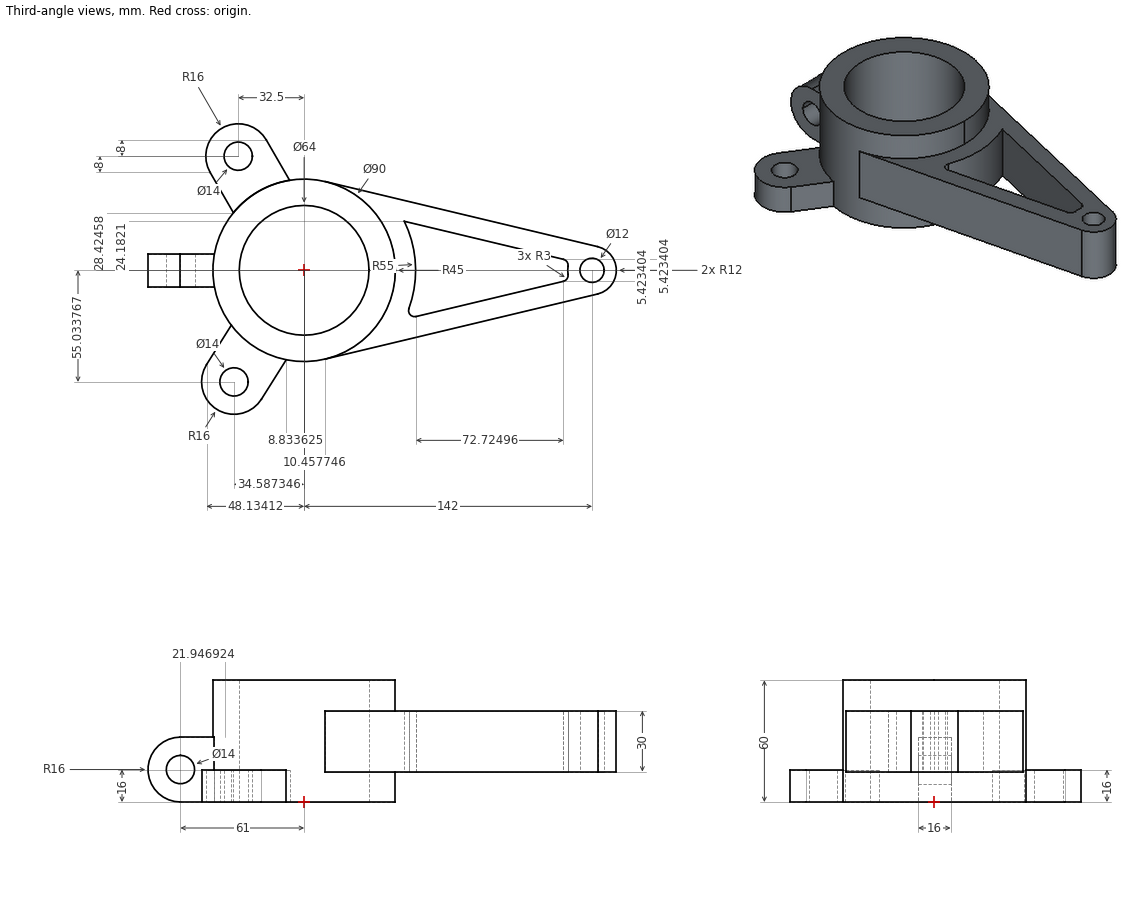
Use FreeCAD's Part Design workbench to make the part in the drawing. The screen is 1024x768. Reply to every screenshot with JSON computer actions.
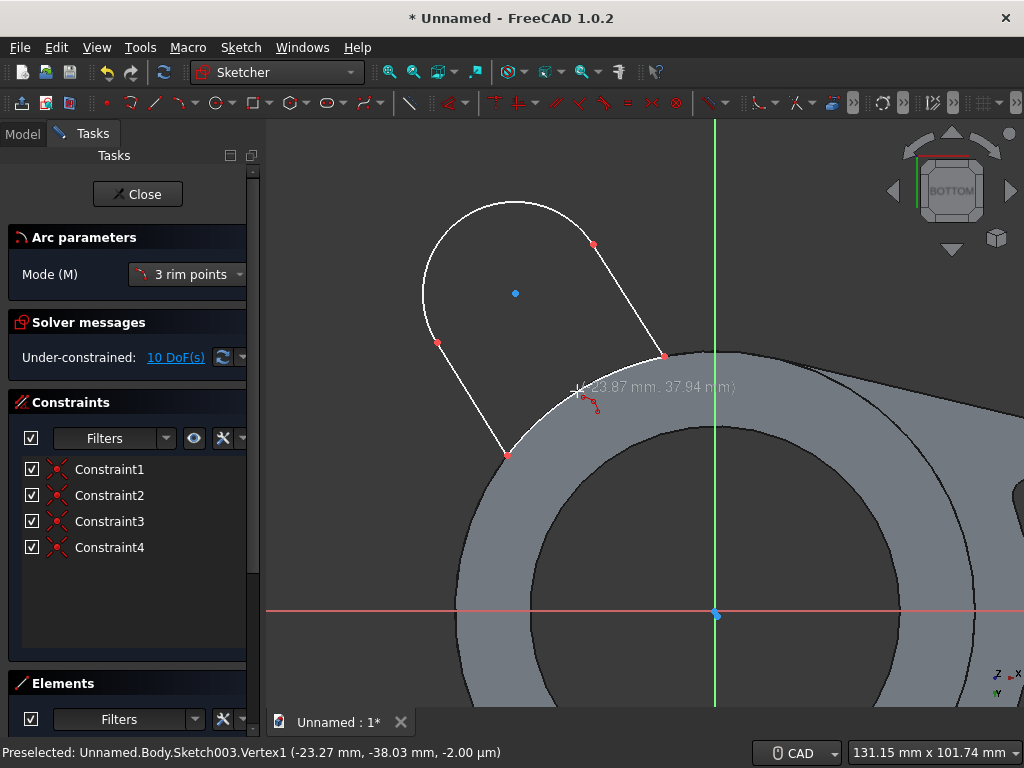
{"action": "left_click", "coordinate": [216, 104]}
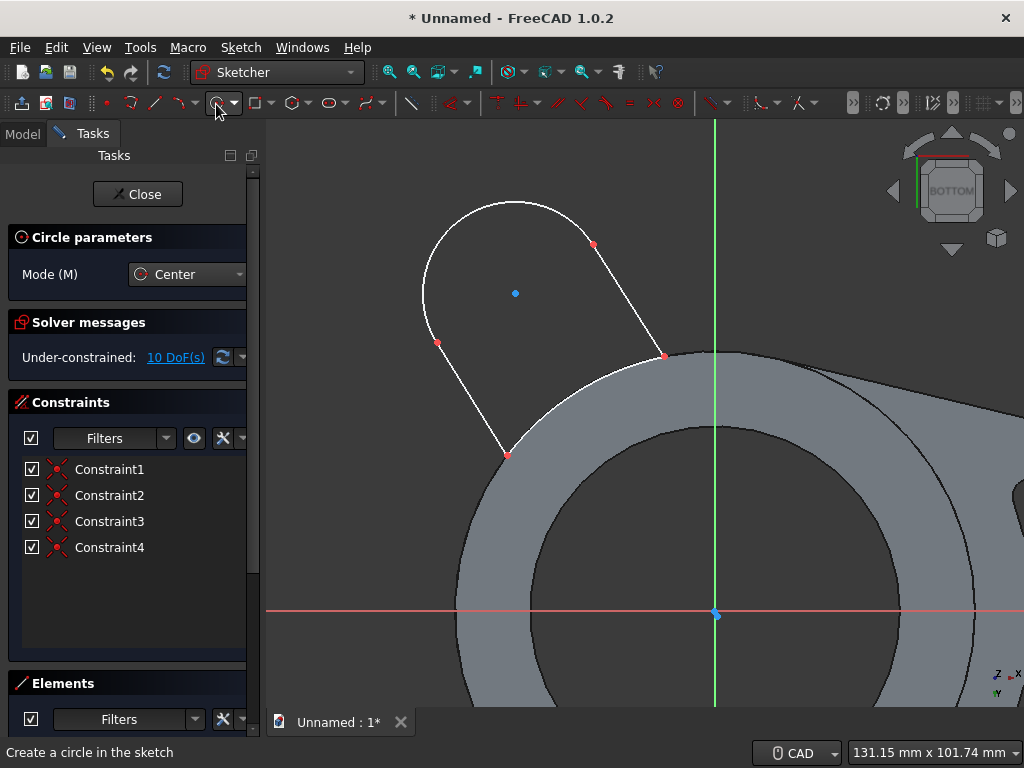
{"action": "left_click", "coordinate": [515, 293]}
{"action": "left_click", "coordinate": [544, 265]}
{"action": "key", "text": "Escape"}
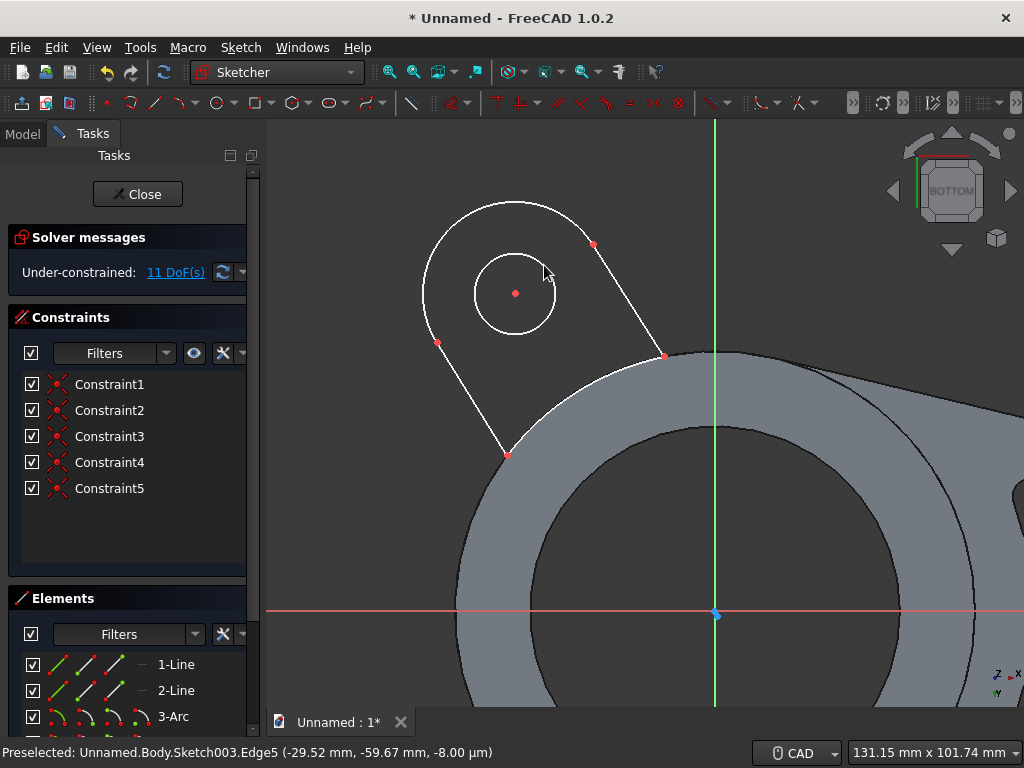
{"action": "left_click", "coordinate": [486, 422]}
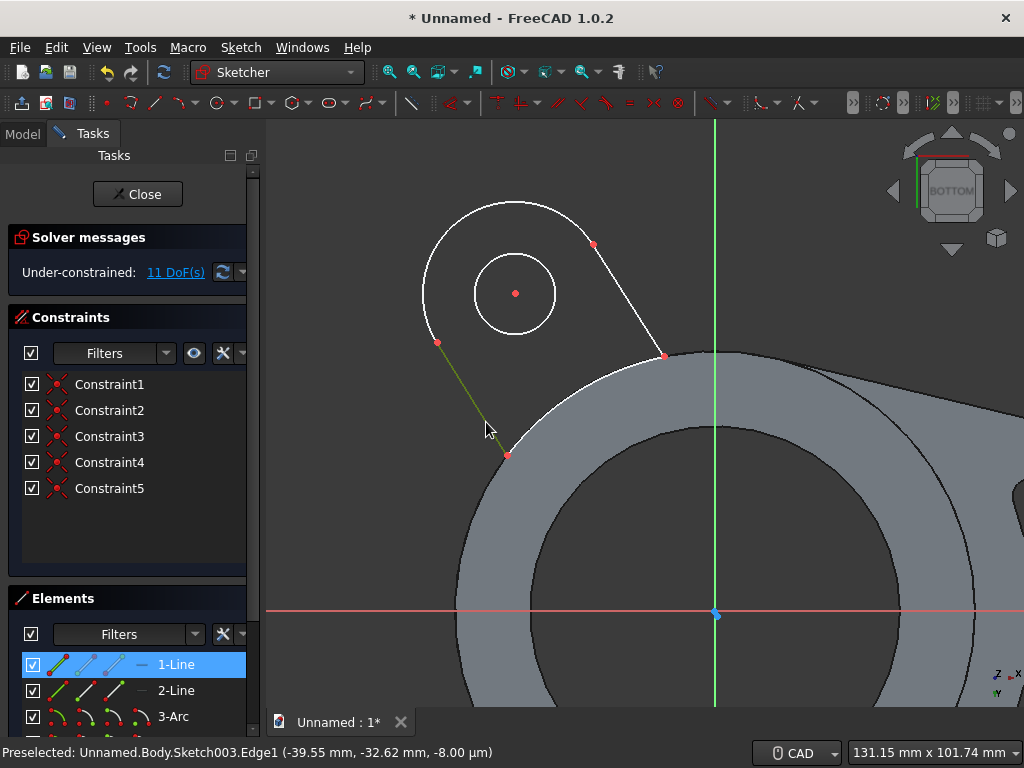
{"action": "left_click", "coordinate": [521, 202]}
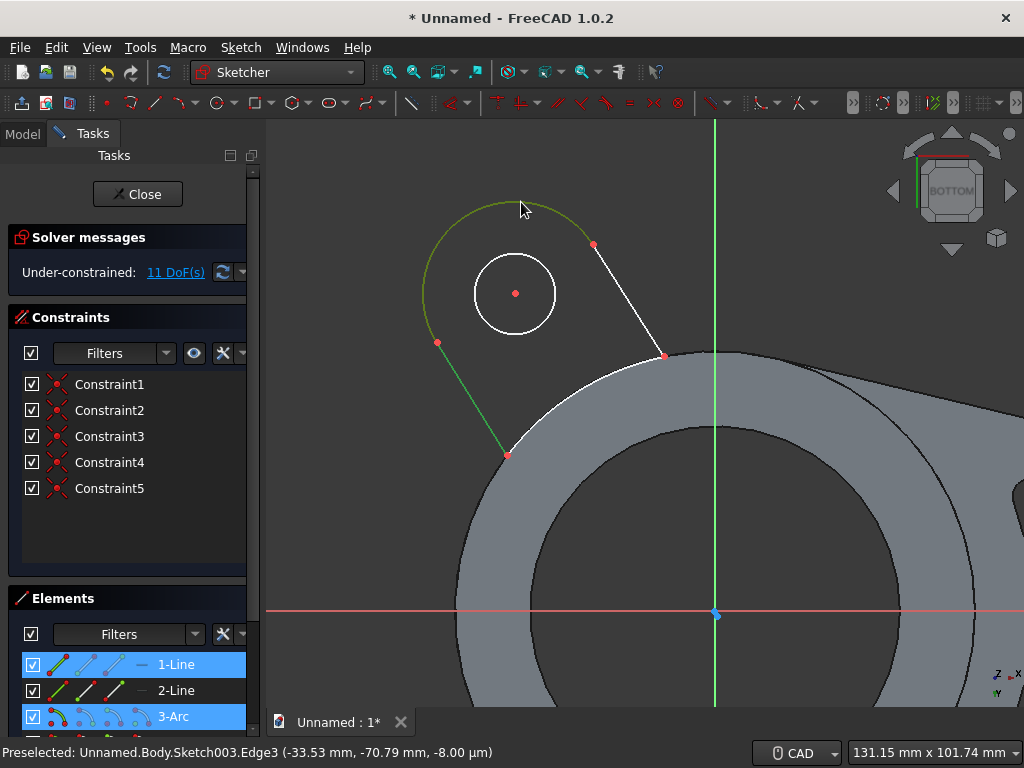
{"action": "key", "text": "t"}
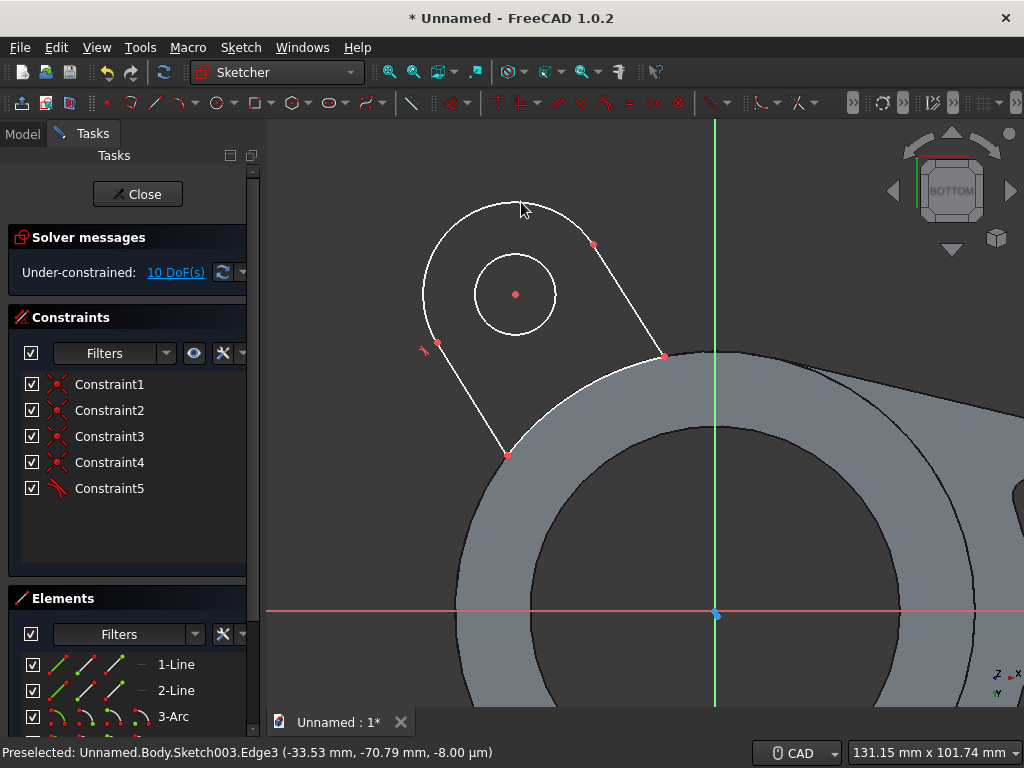
{"action": "left_click", "coordinate": [614, 279]}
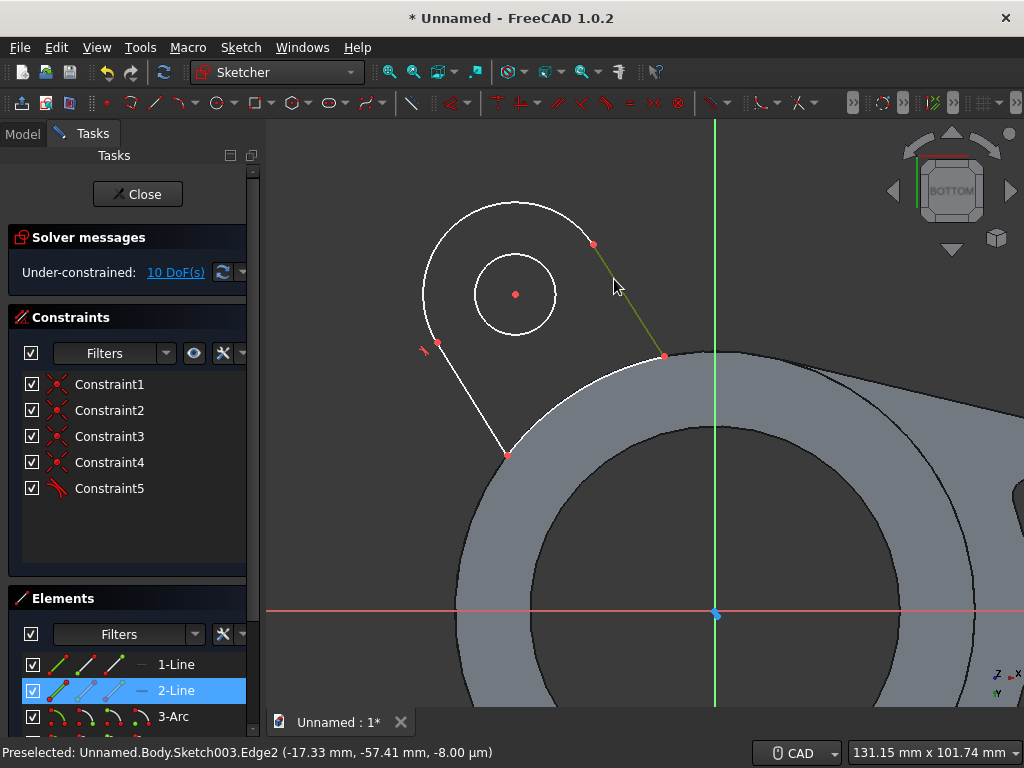
{"action": "left_click", "coordinate": [521, 203]}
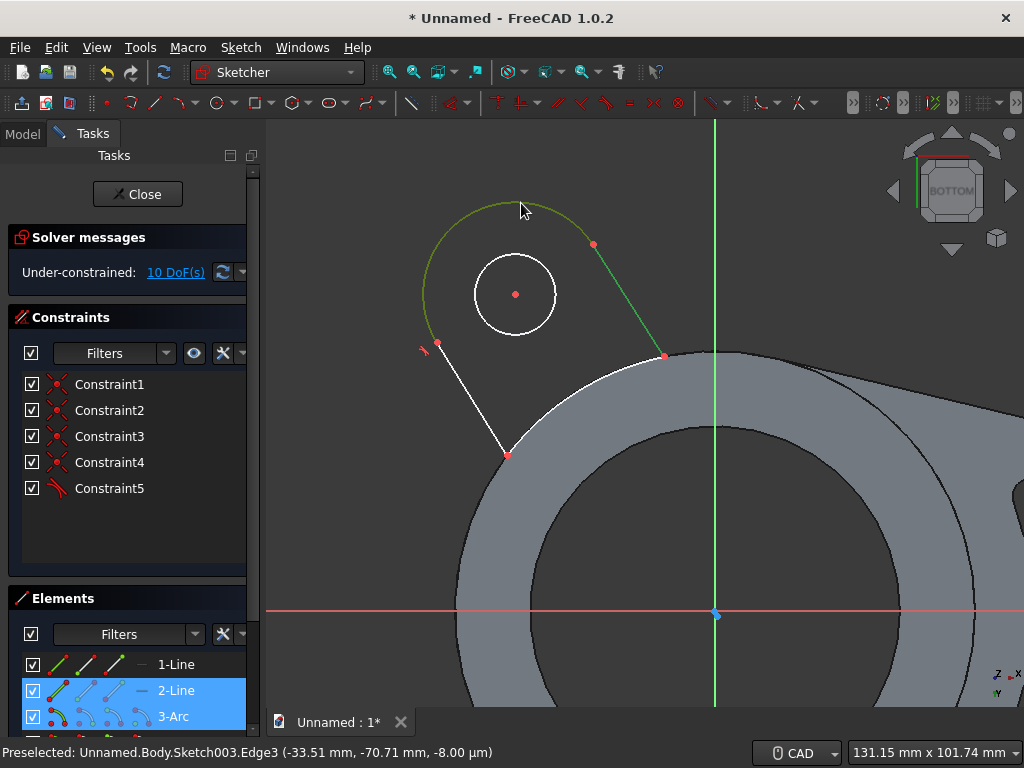
{"action": "left_click", "coordinate": [606, 104]}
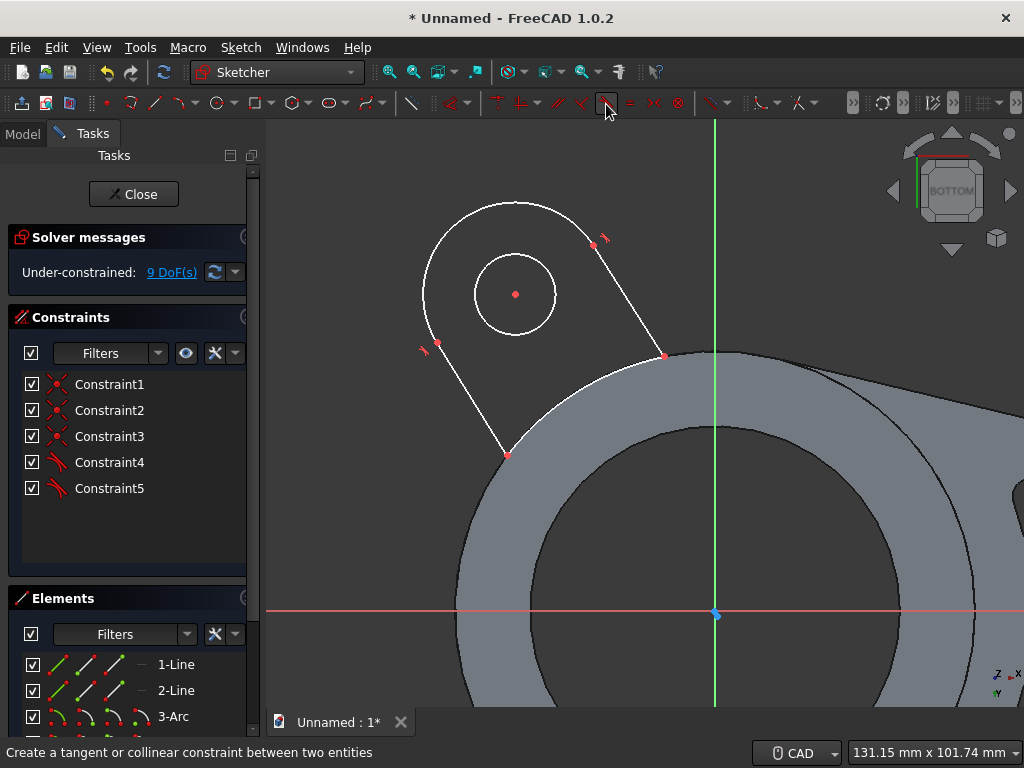
{"action": "left_click_drag", "start_coordinate": [705, 601], "coordinate": [728, 626]}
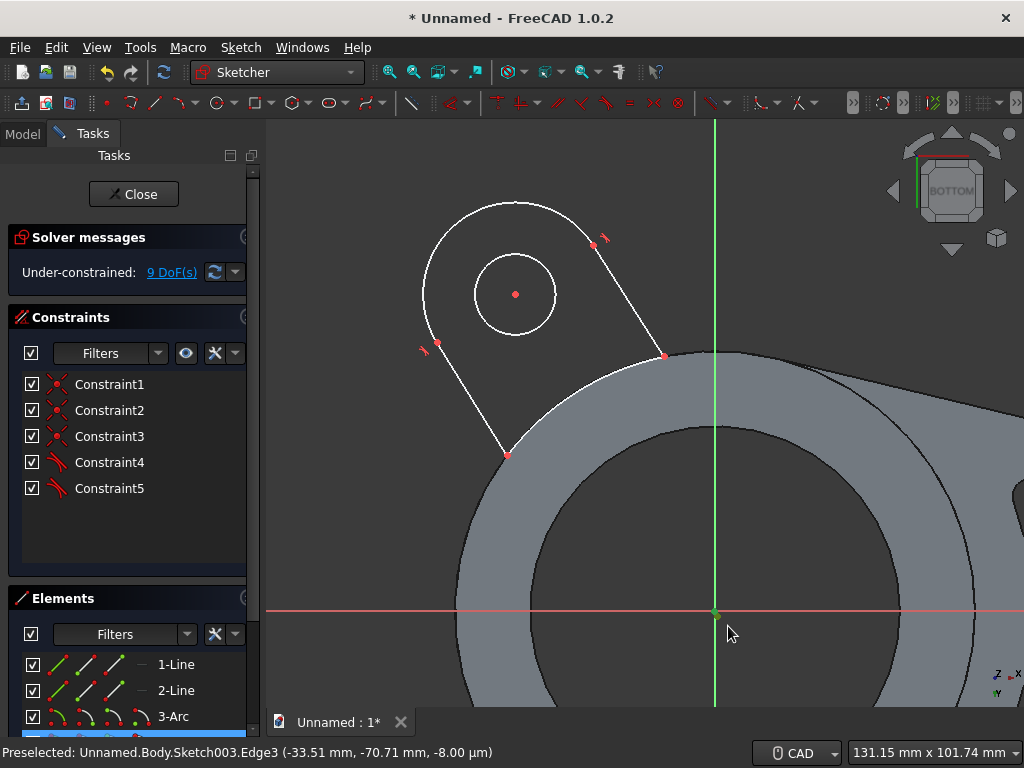
{"action": "key", "text": "c"}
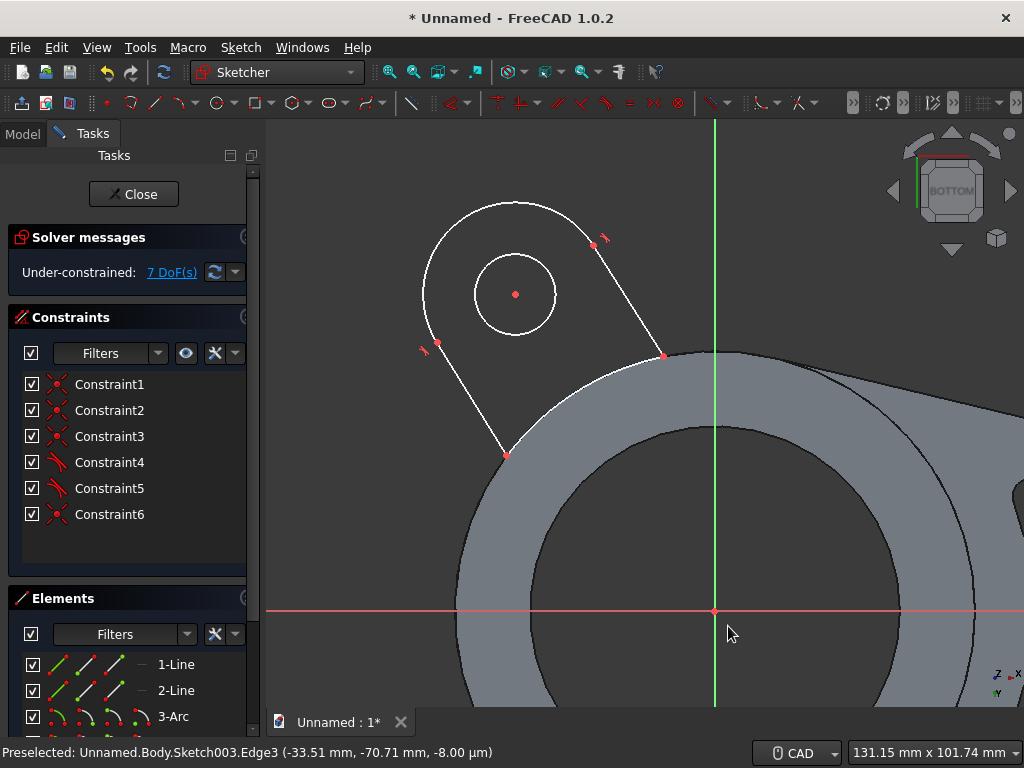
{"action": "key", "text": "d"}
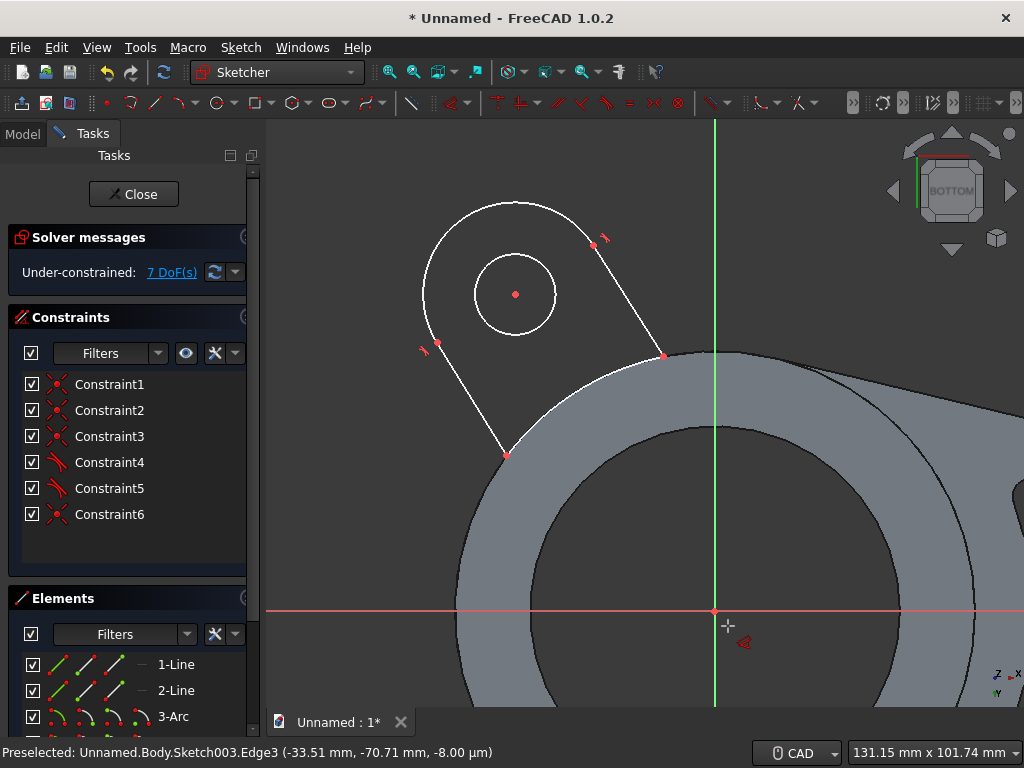
{"action": "left_click", "coordinate": [521, 203]}
{"action": "left_click", "coordinate": [523, 171]}